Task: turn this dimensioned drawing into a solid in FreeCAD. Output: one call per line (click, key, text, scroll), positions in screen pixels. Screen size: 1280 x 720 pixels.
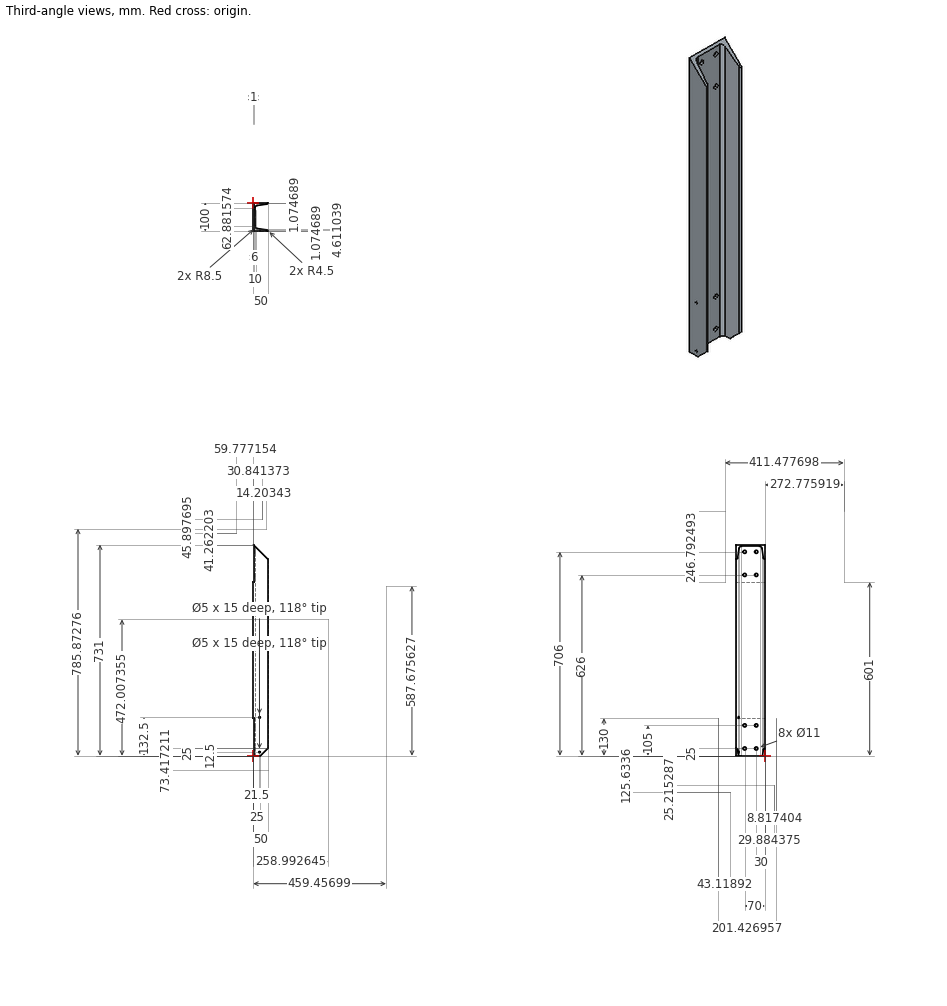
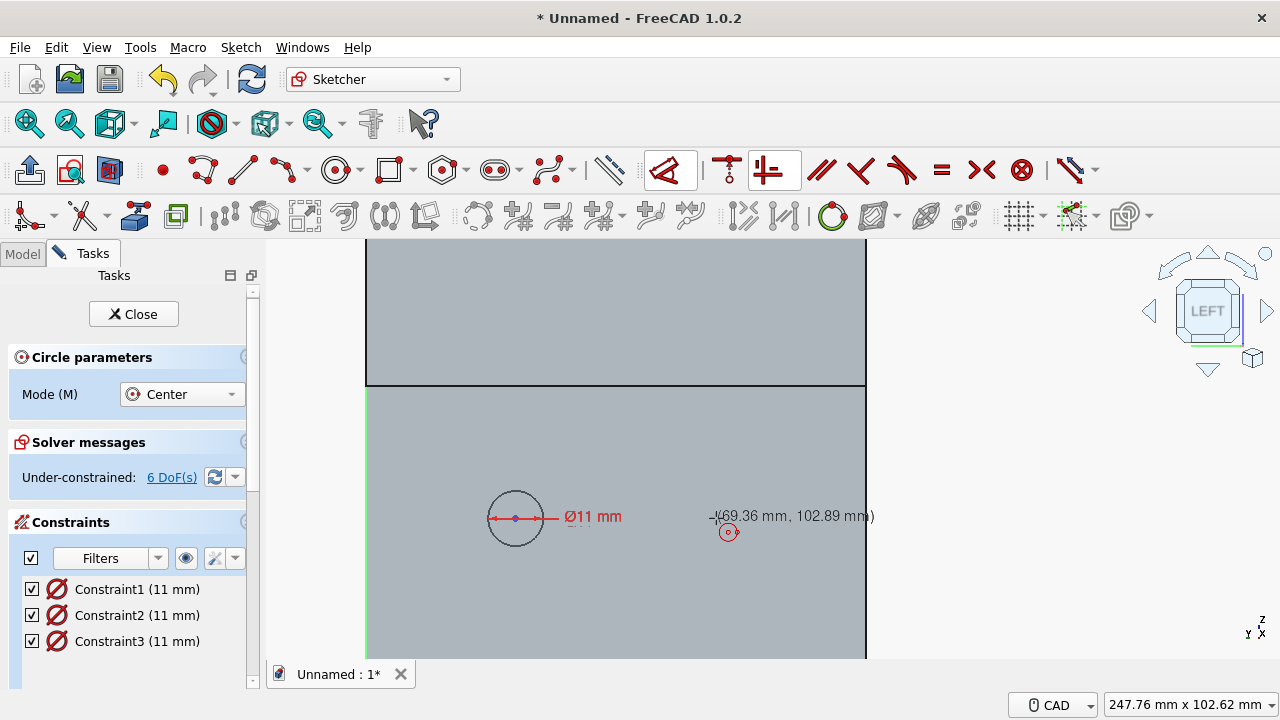
scroll(716, 545, down, 13)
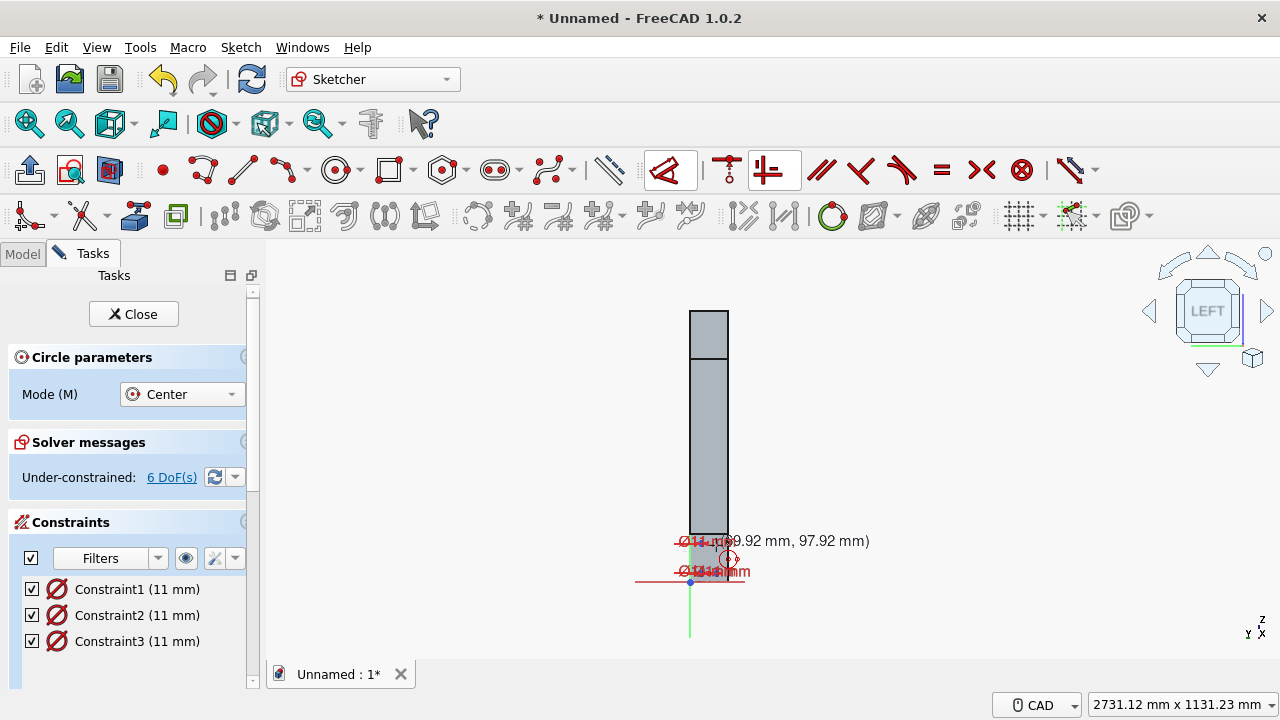
scroll(716, 543, up, 2)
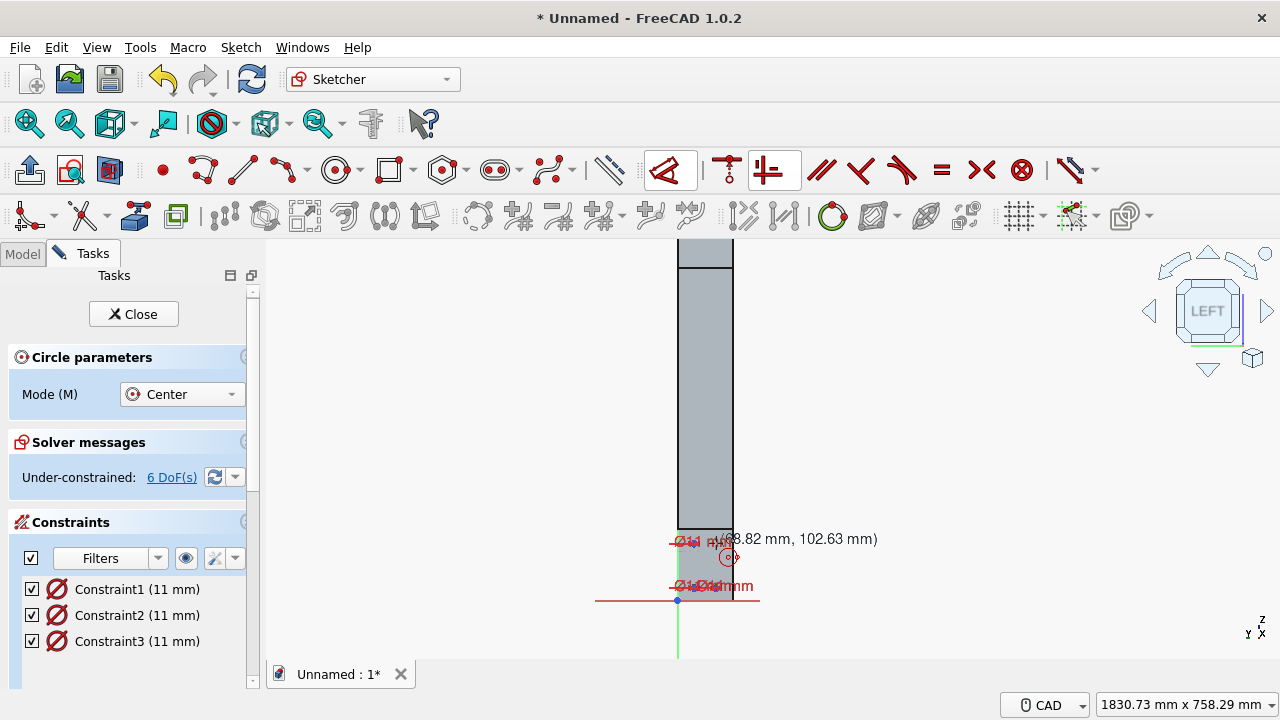
click(716, 543)
move(719, 541)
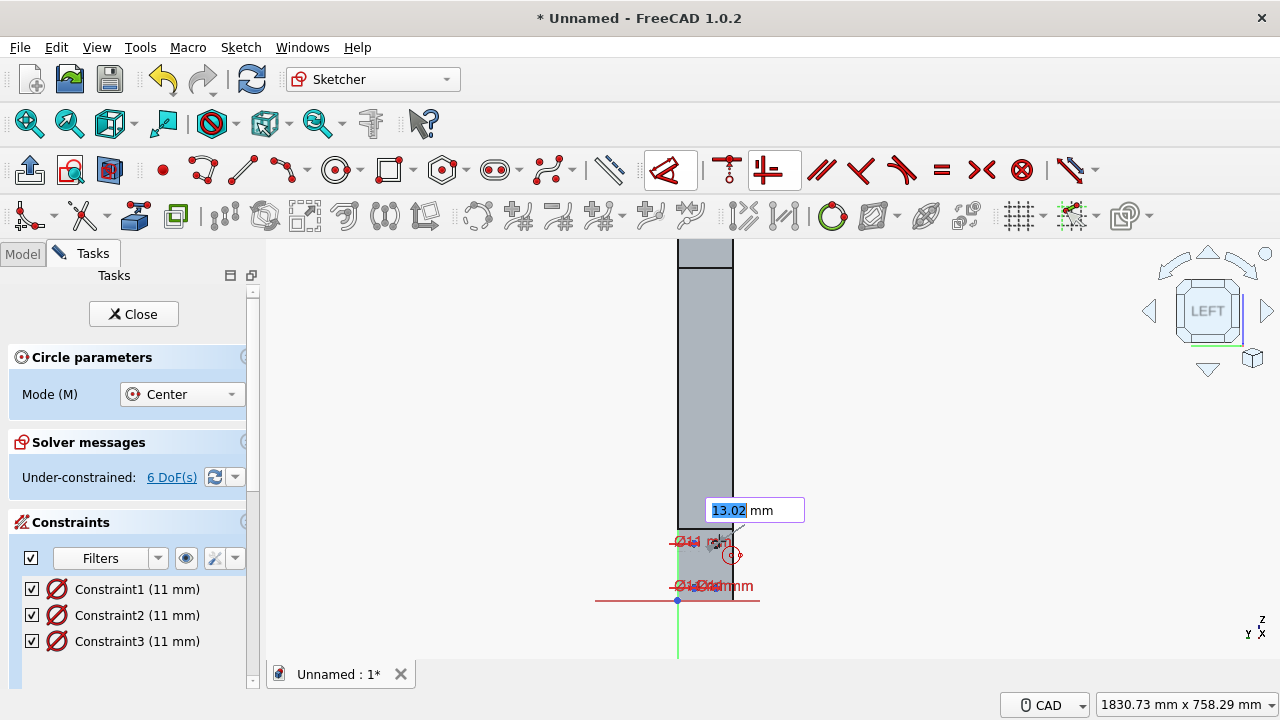
text(11)
key(Return)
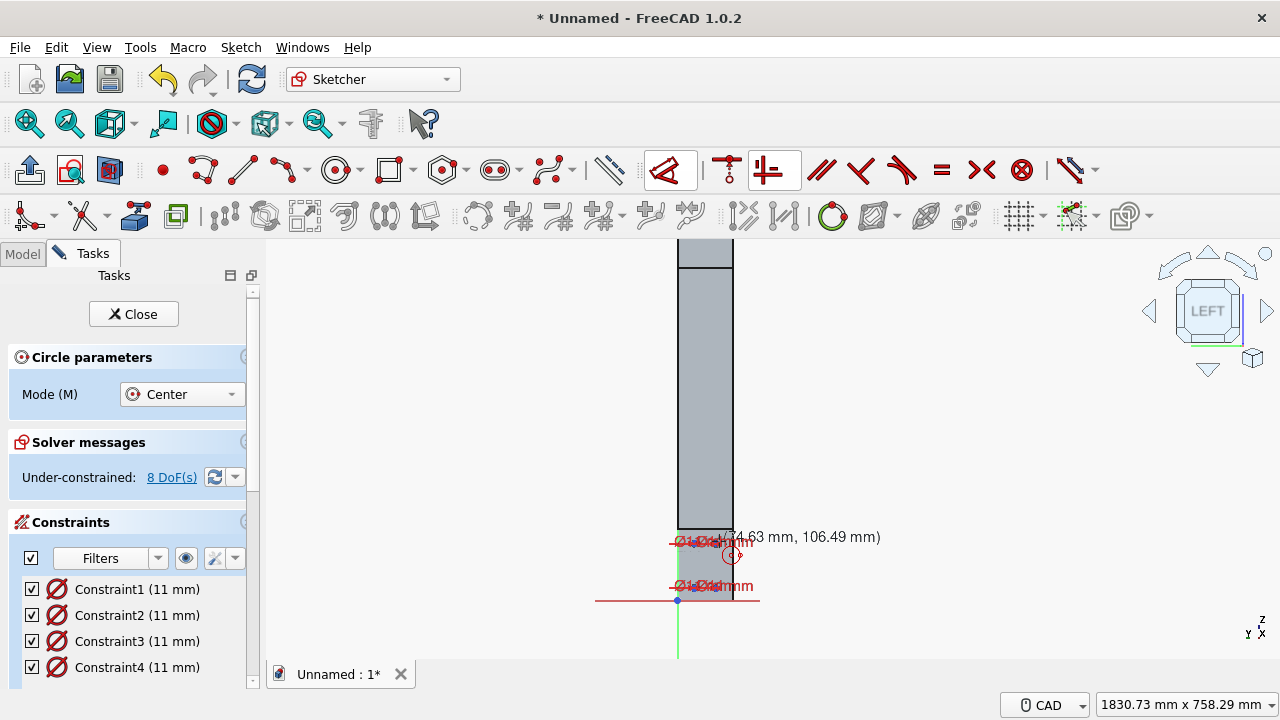
scroll(717, 541, down, 2)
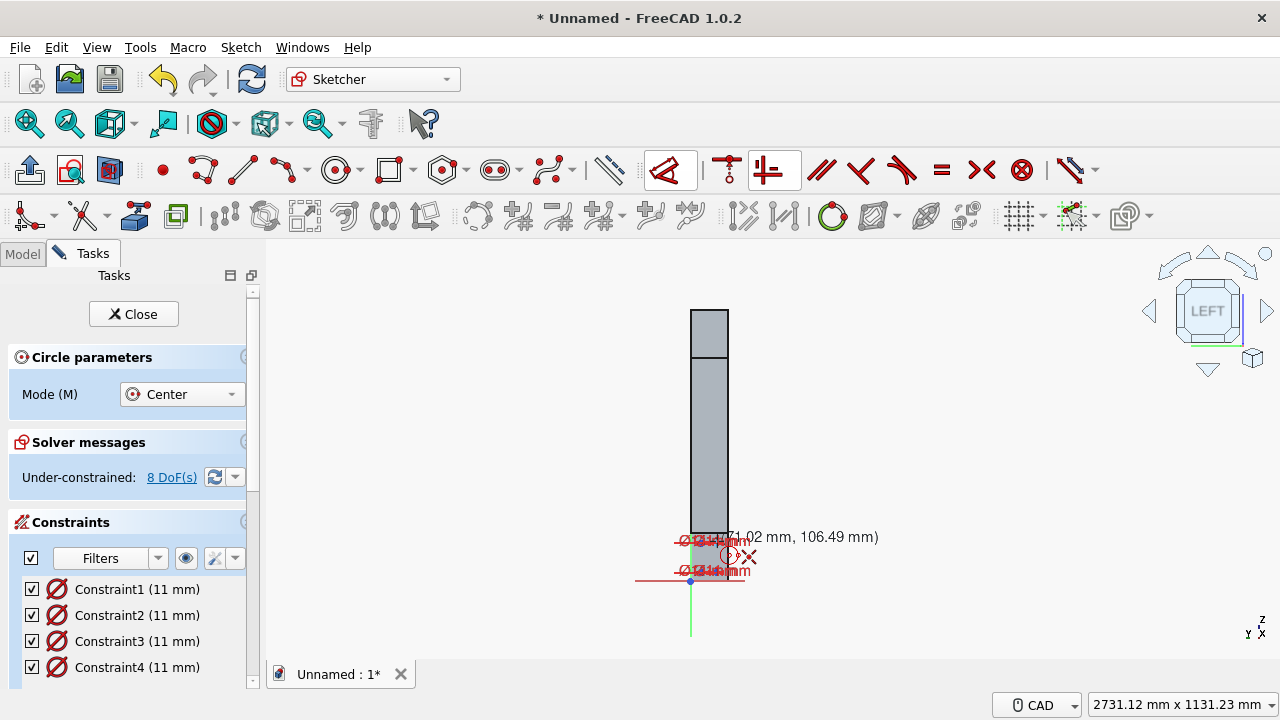
scroll(702, 349, up, 13)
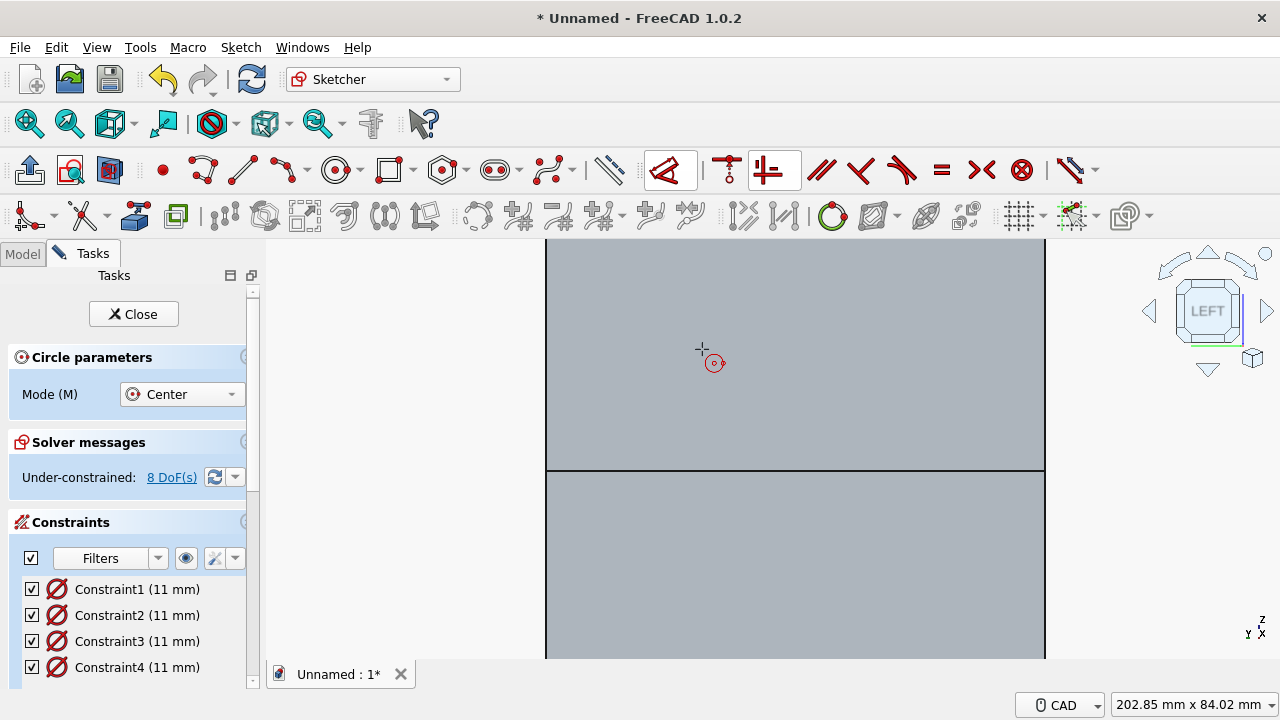
scroll(702, 349, down, 13)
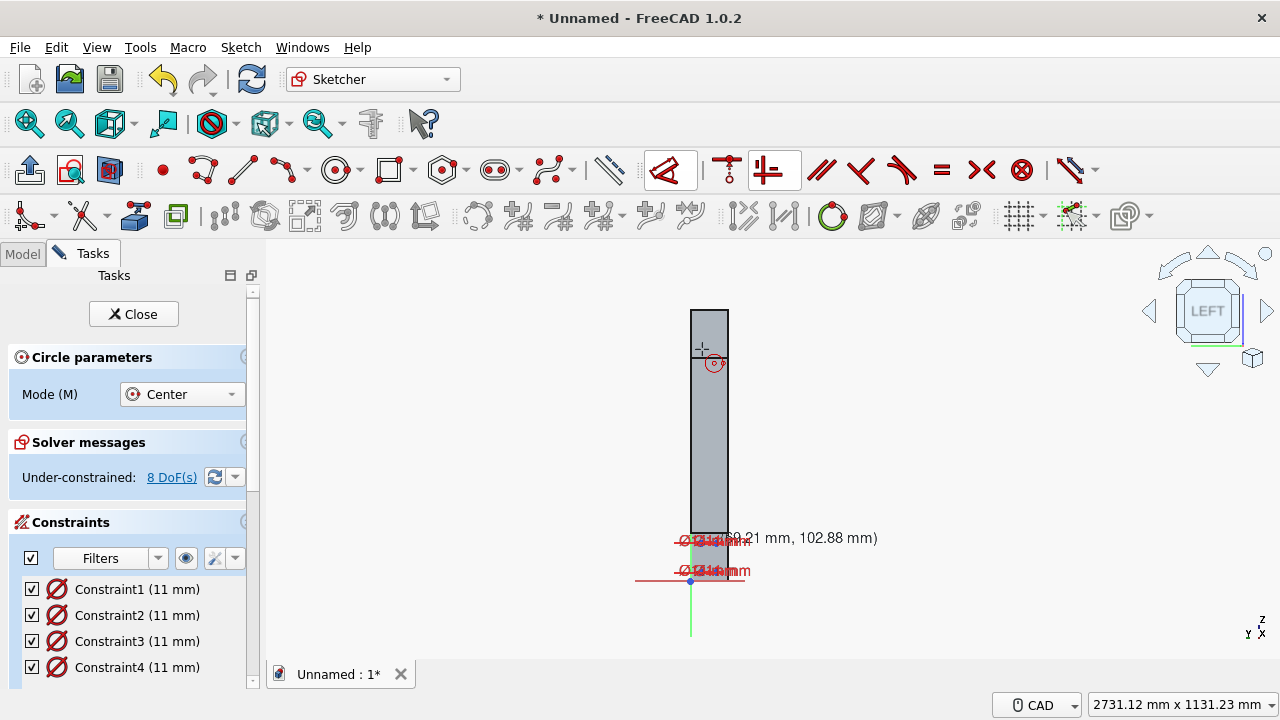
scroll(702, 349, up, 2)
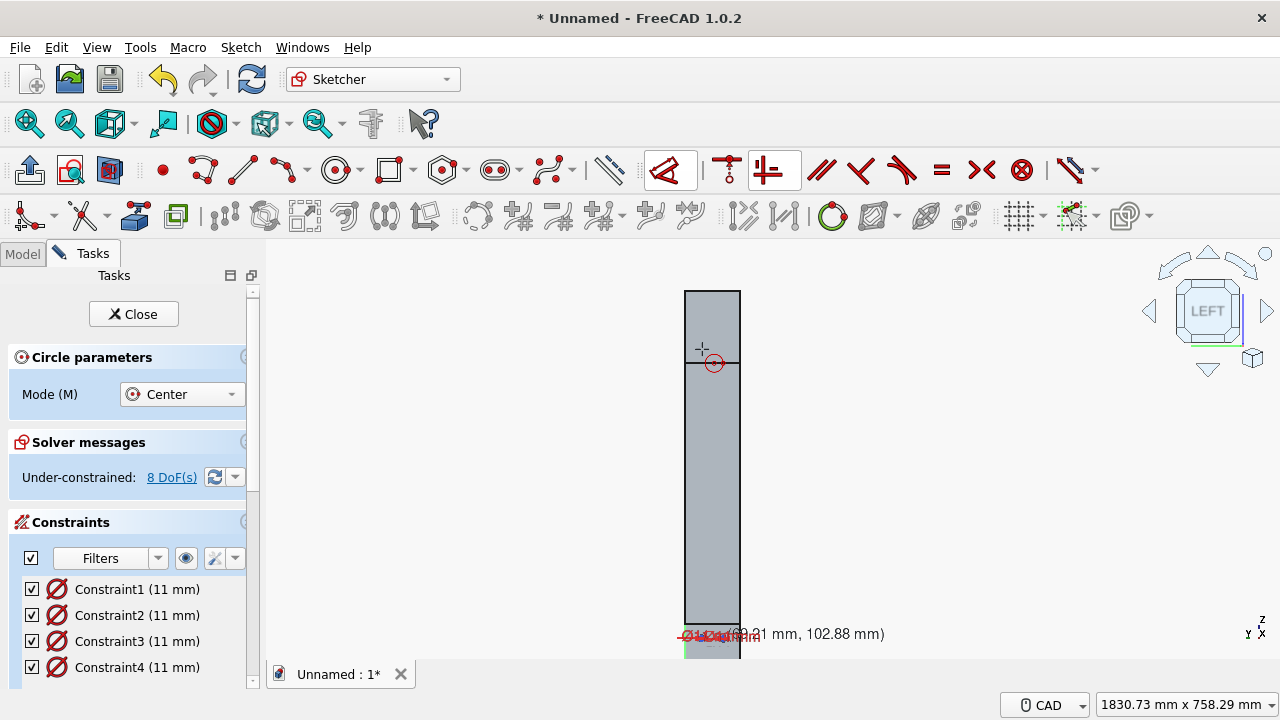
click(702, 349)
move(704, 347)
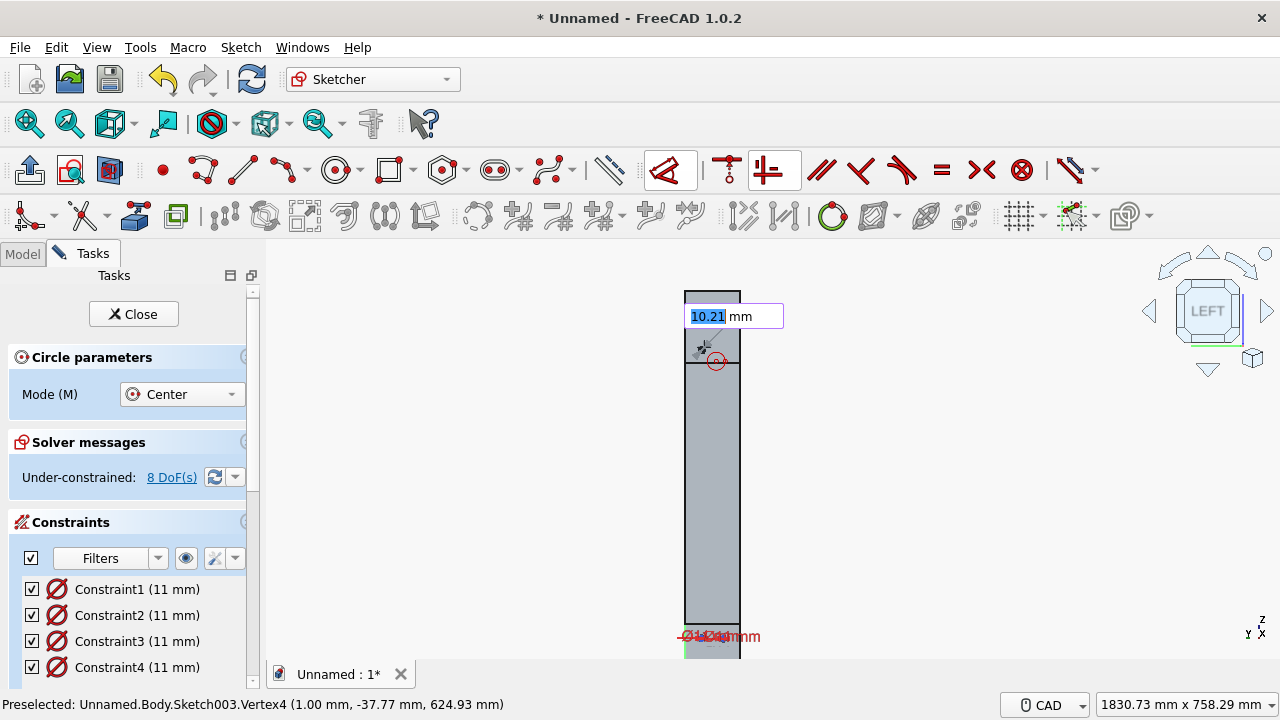
text(11)
key(Return)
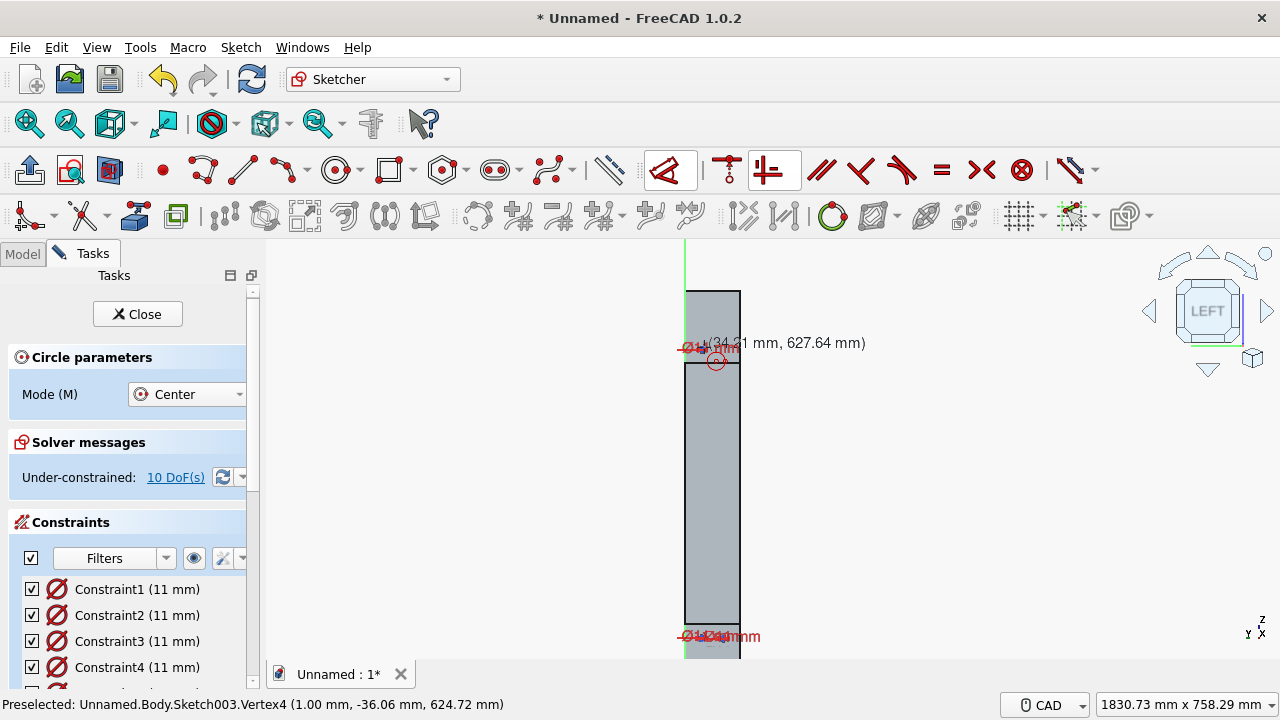
scroll(724, 305, up, 11)